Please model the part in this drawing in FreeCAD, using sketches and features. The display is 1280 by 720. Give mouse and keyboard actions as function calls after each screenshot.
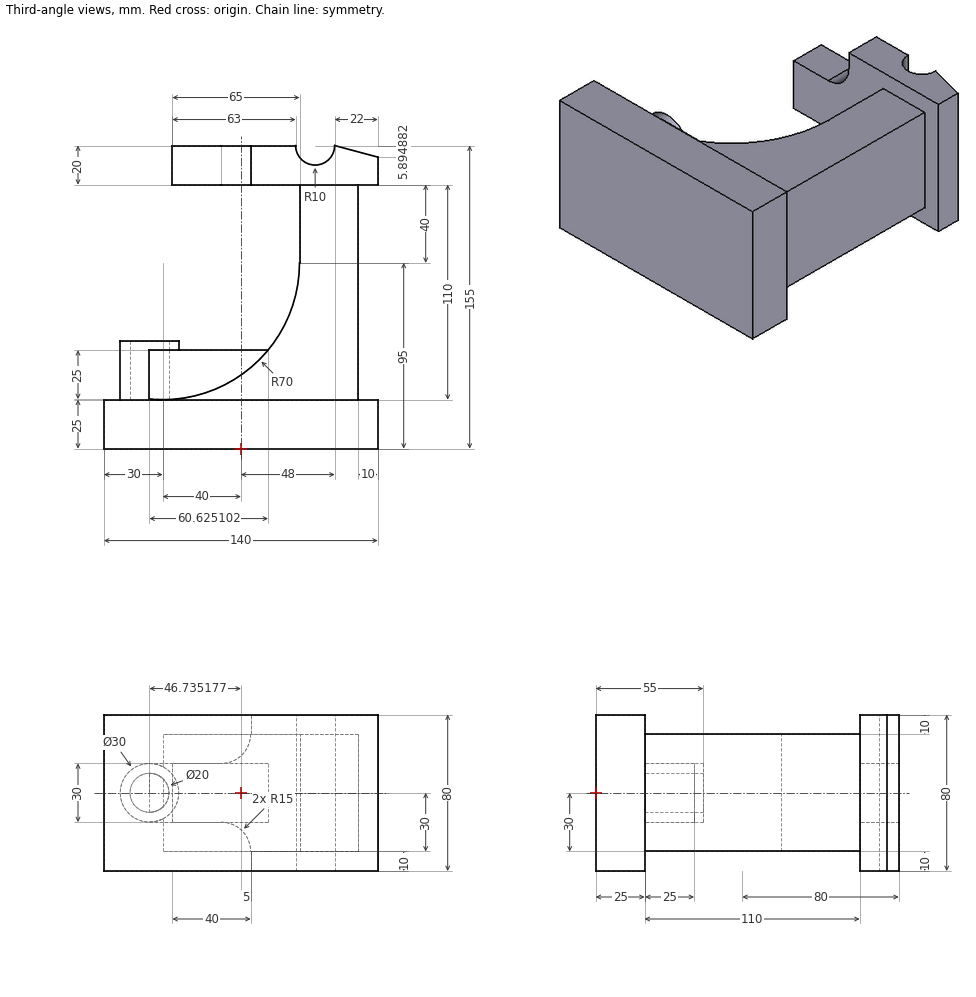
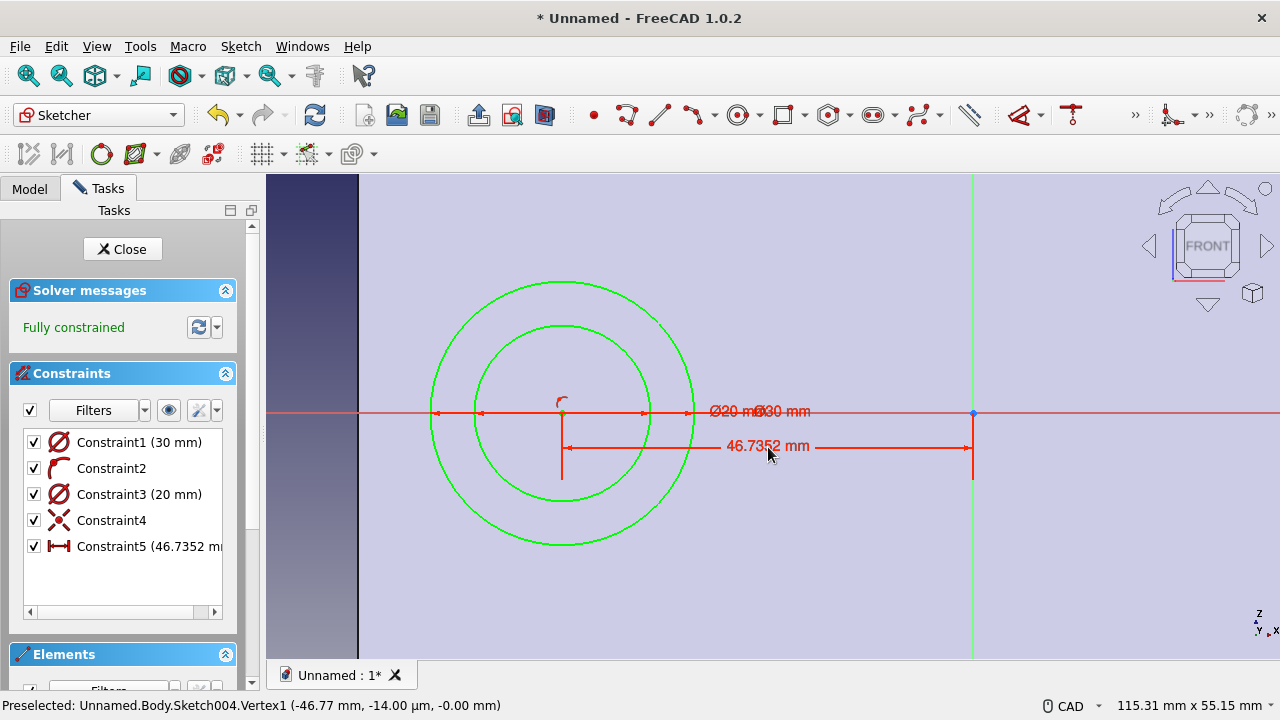
click(123, 249)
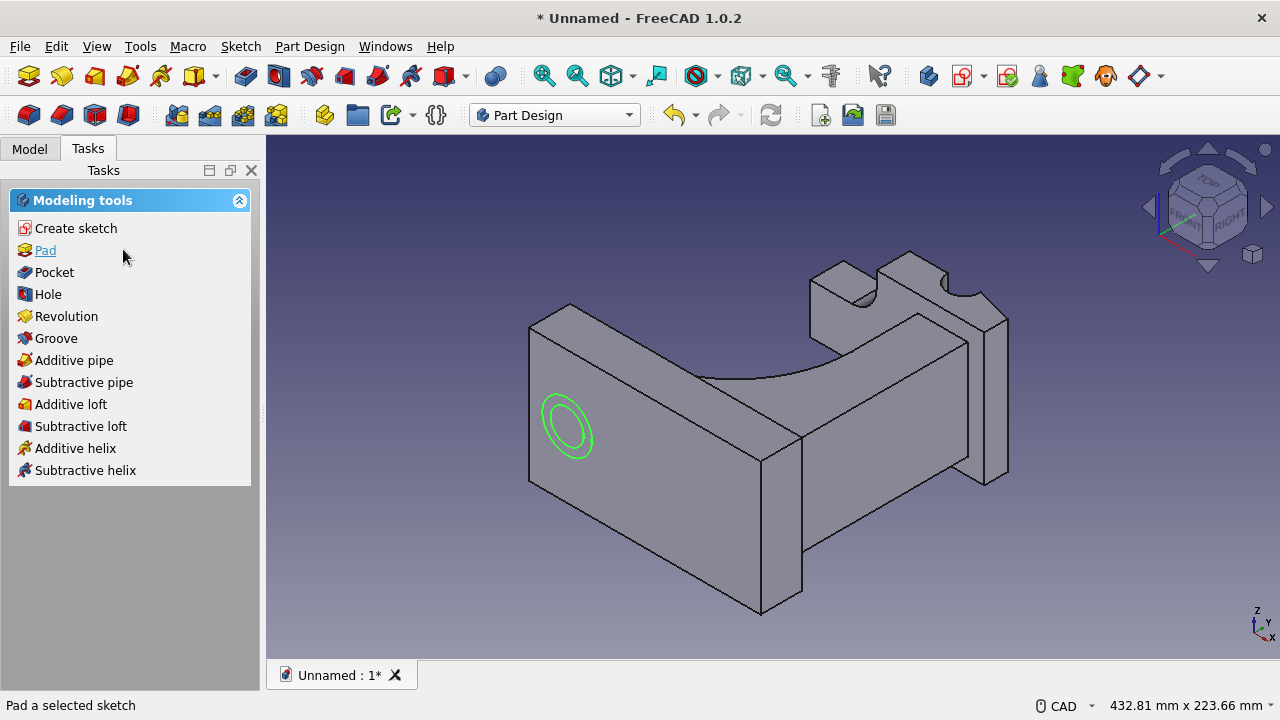
click(29, 76)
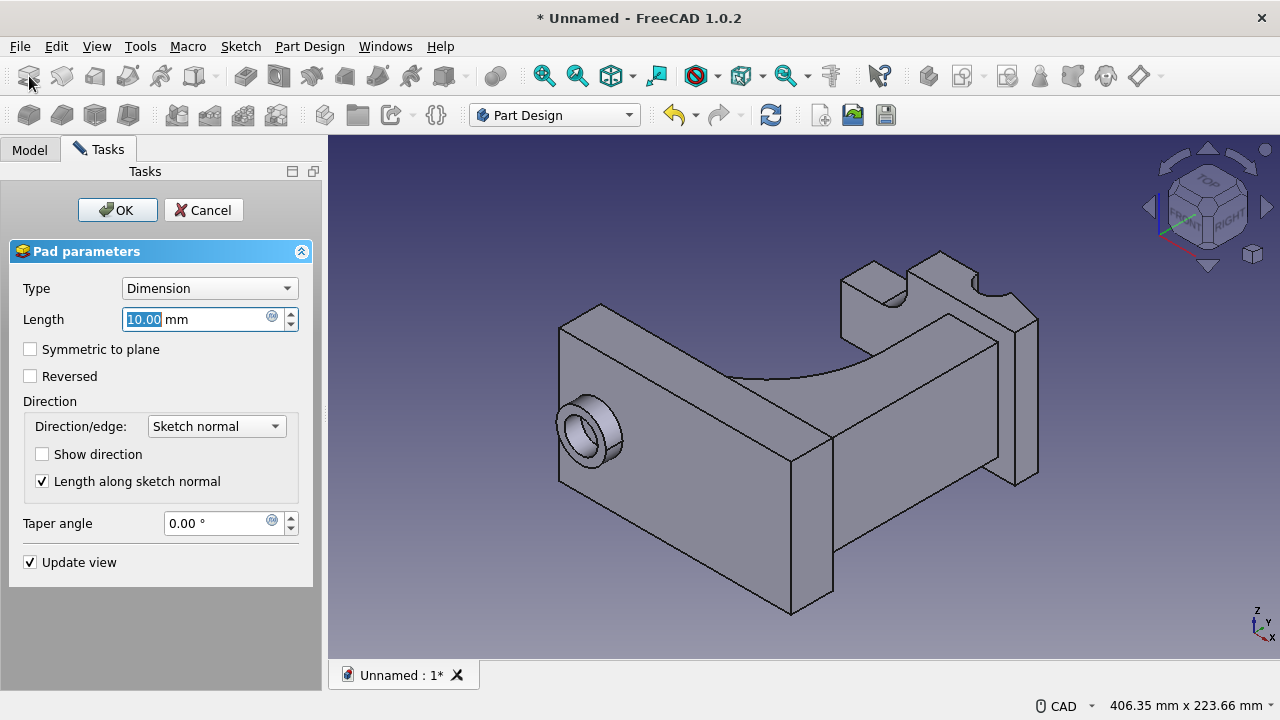
text(55)
key(Tab)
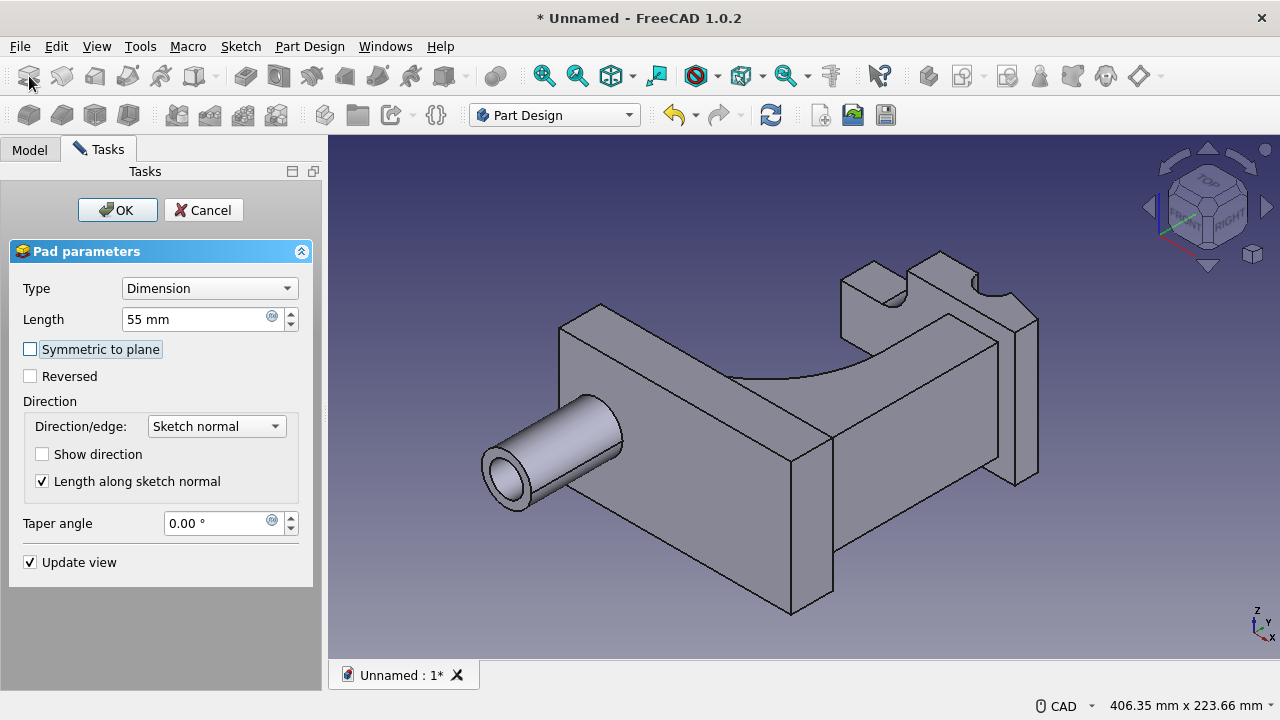
click(31, 376)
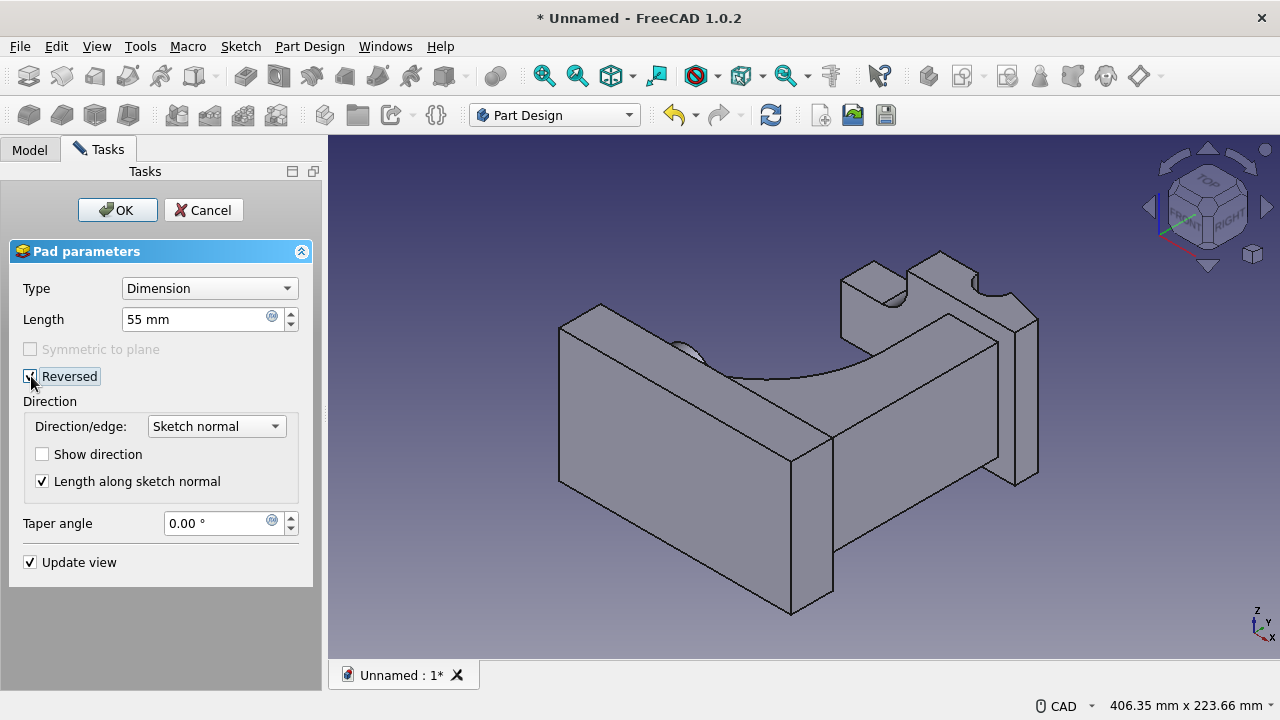
click(118, 210)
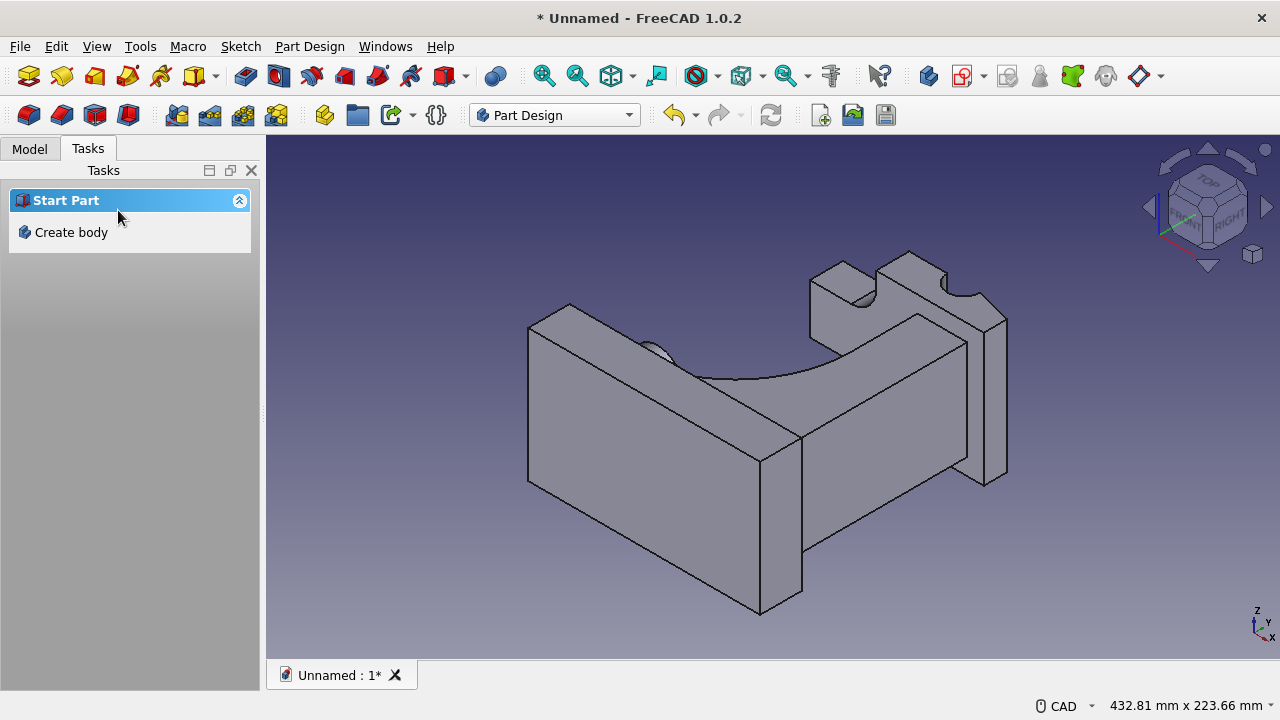
click(962, 76)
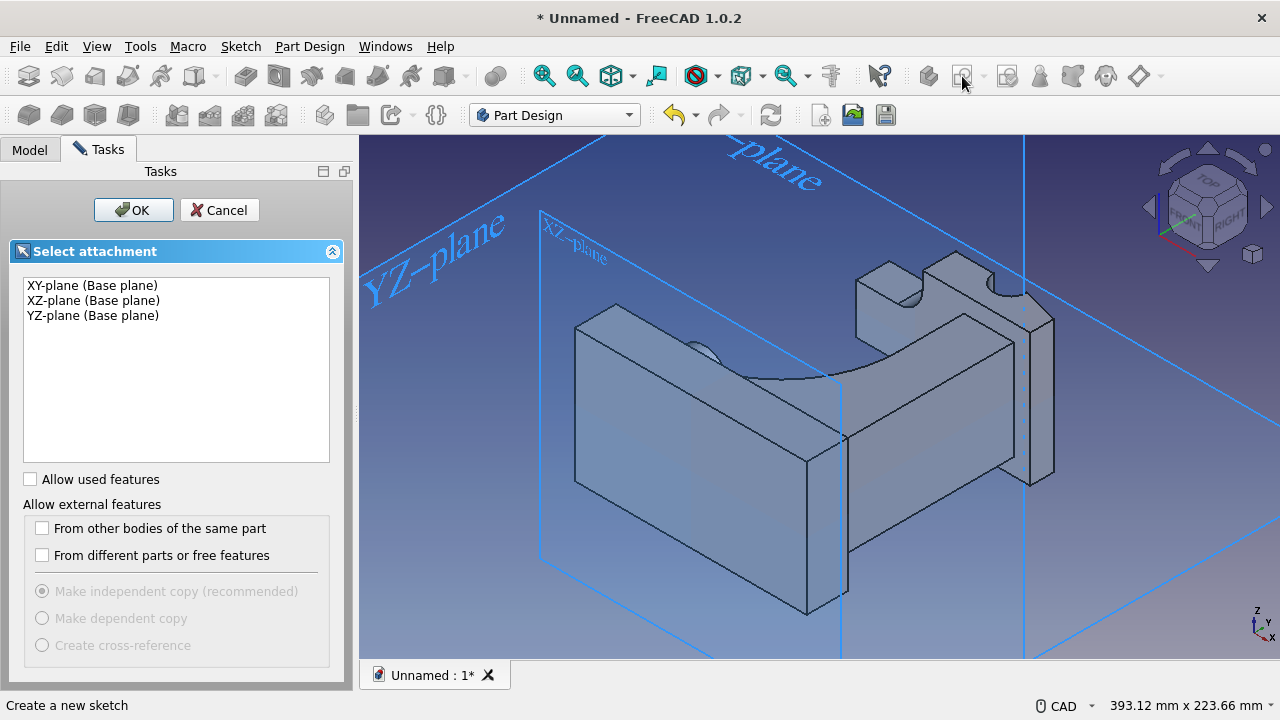
click(84, 286)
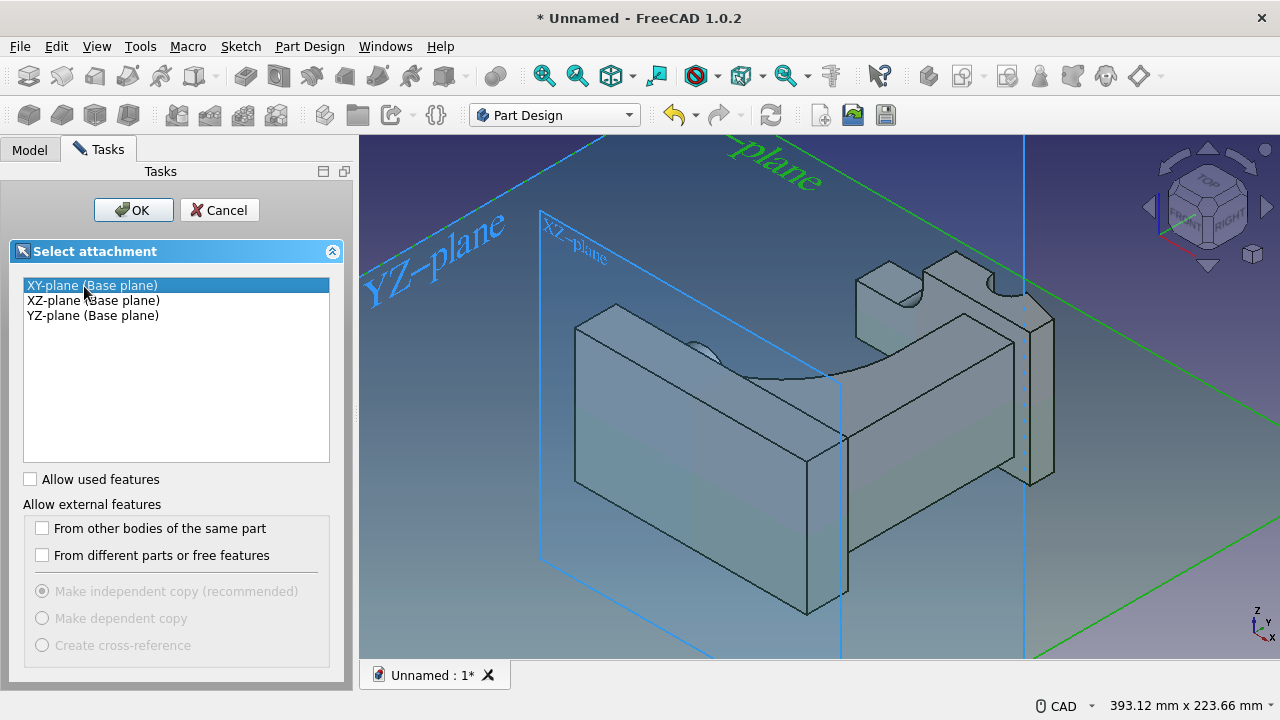
click(134, 210)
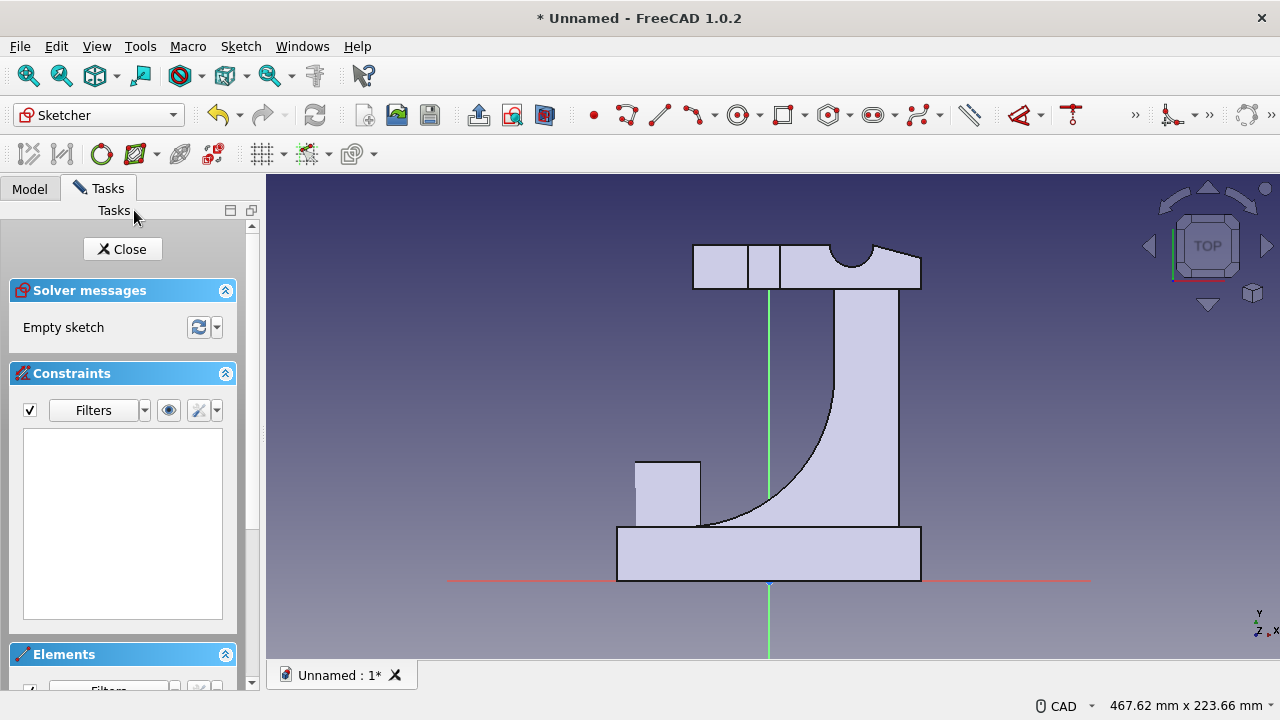
click(545, 116)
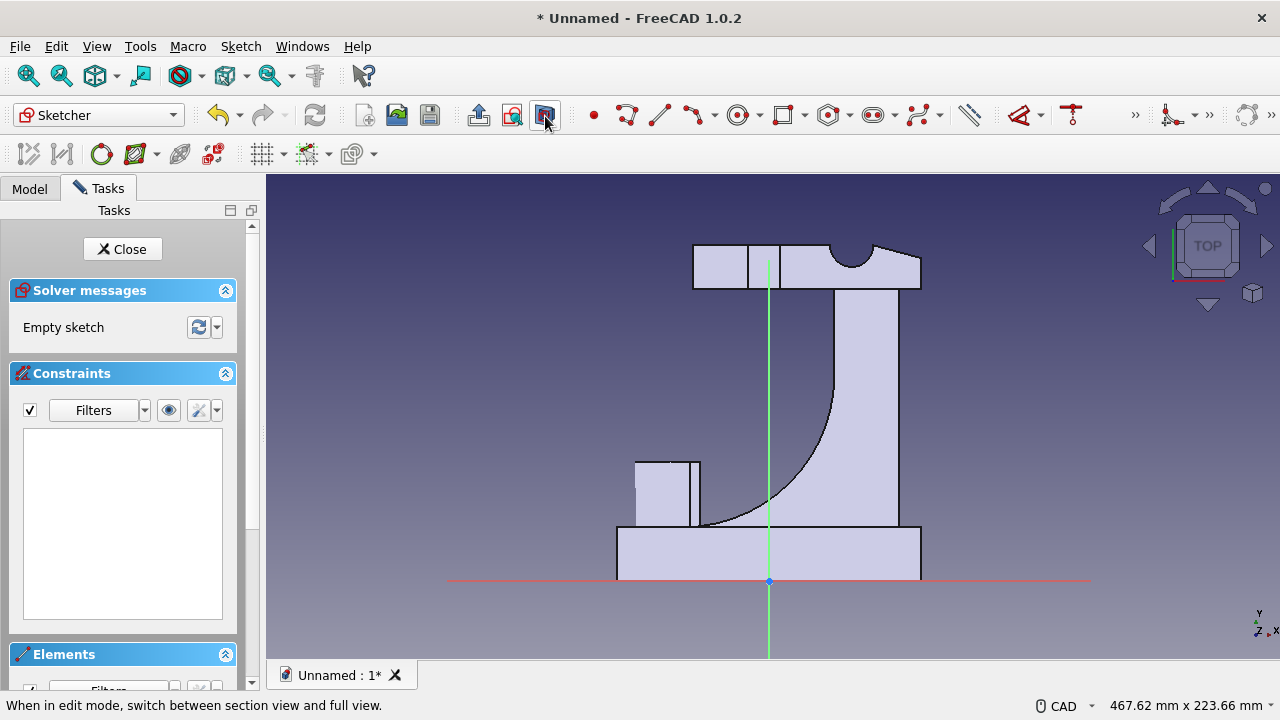
scroll(751, 591, up, 5)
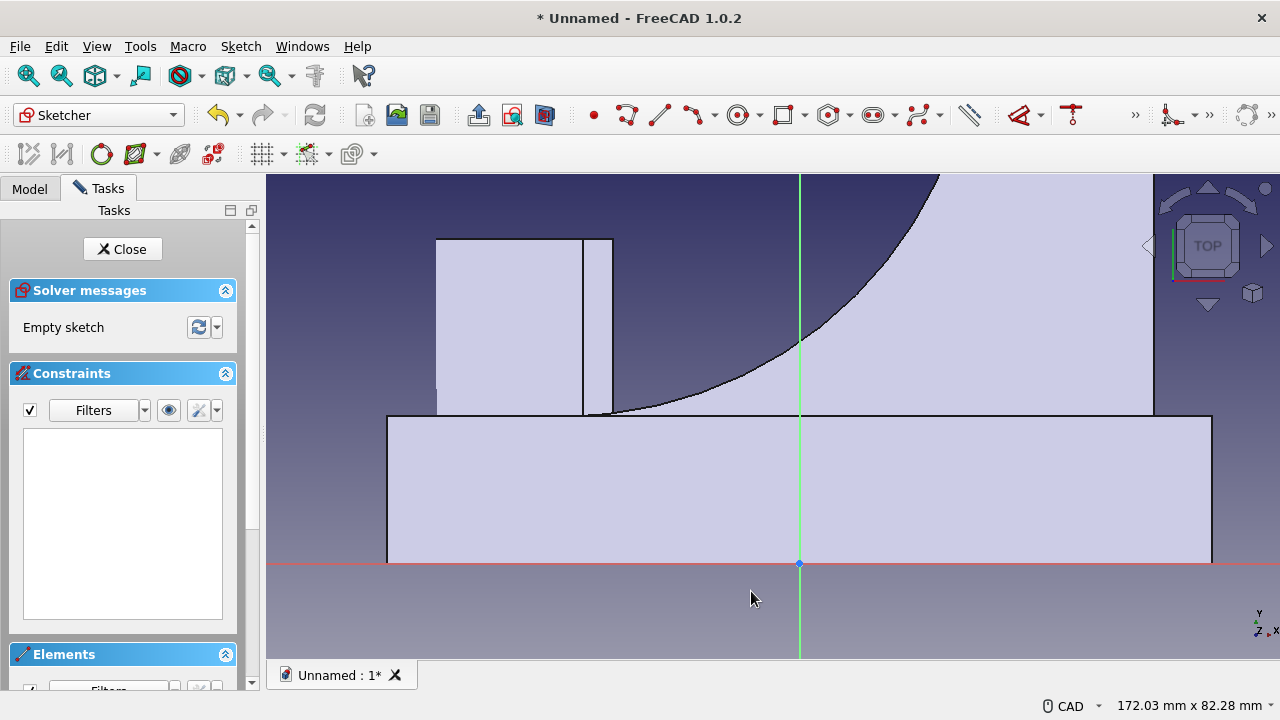
click(627, 116)